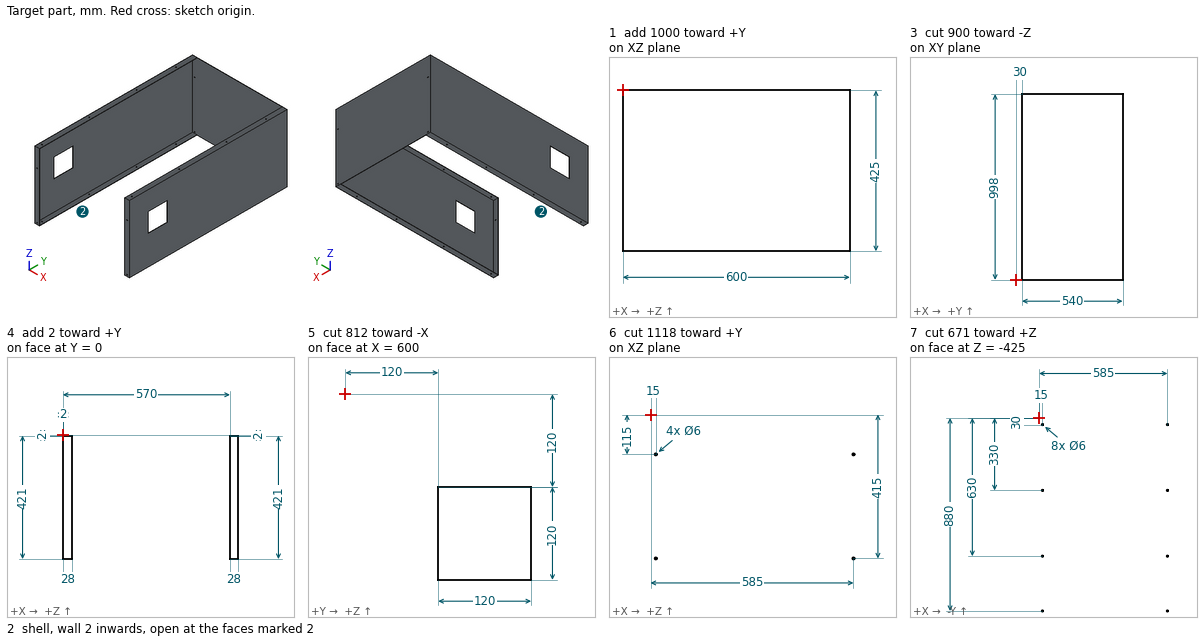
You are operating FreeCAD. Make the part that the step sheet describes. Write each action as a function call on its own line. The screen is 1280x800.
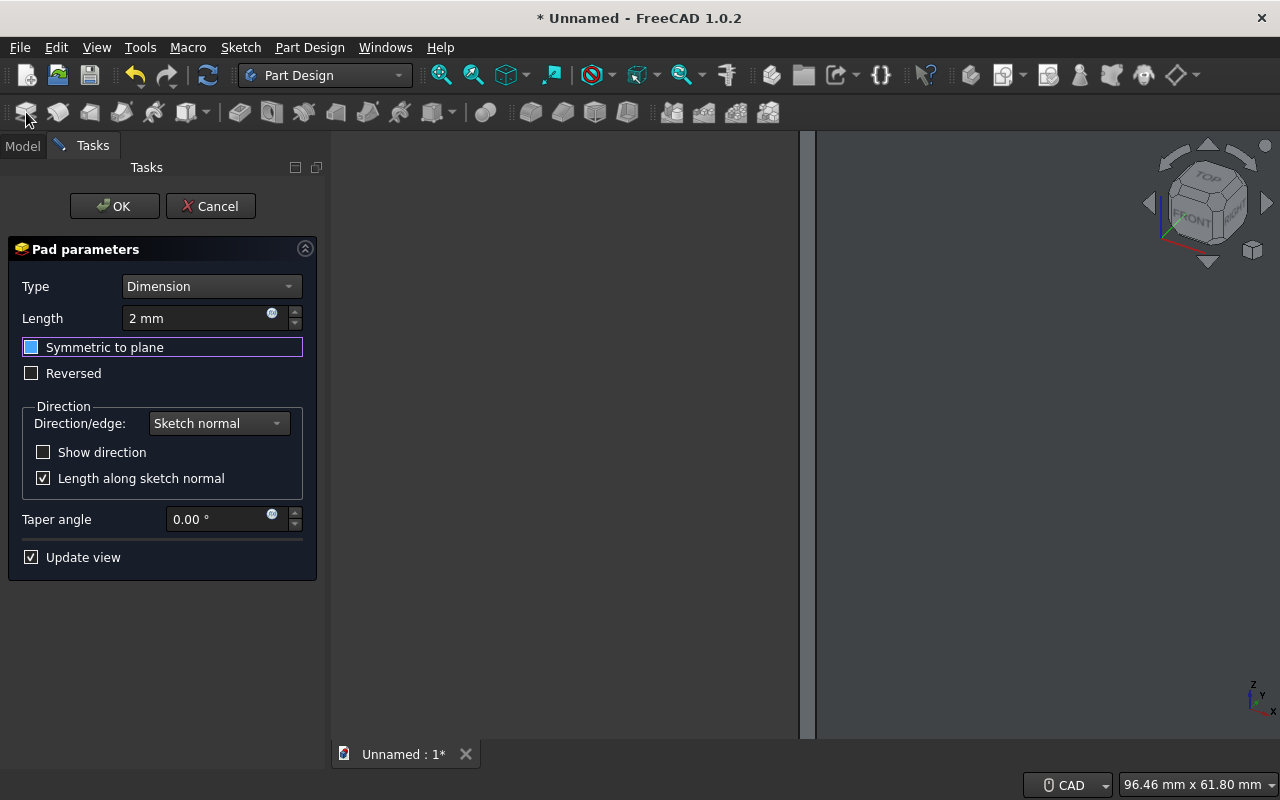
click(30, 373)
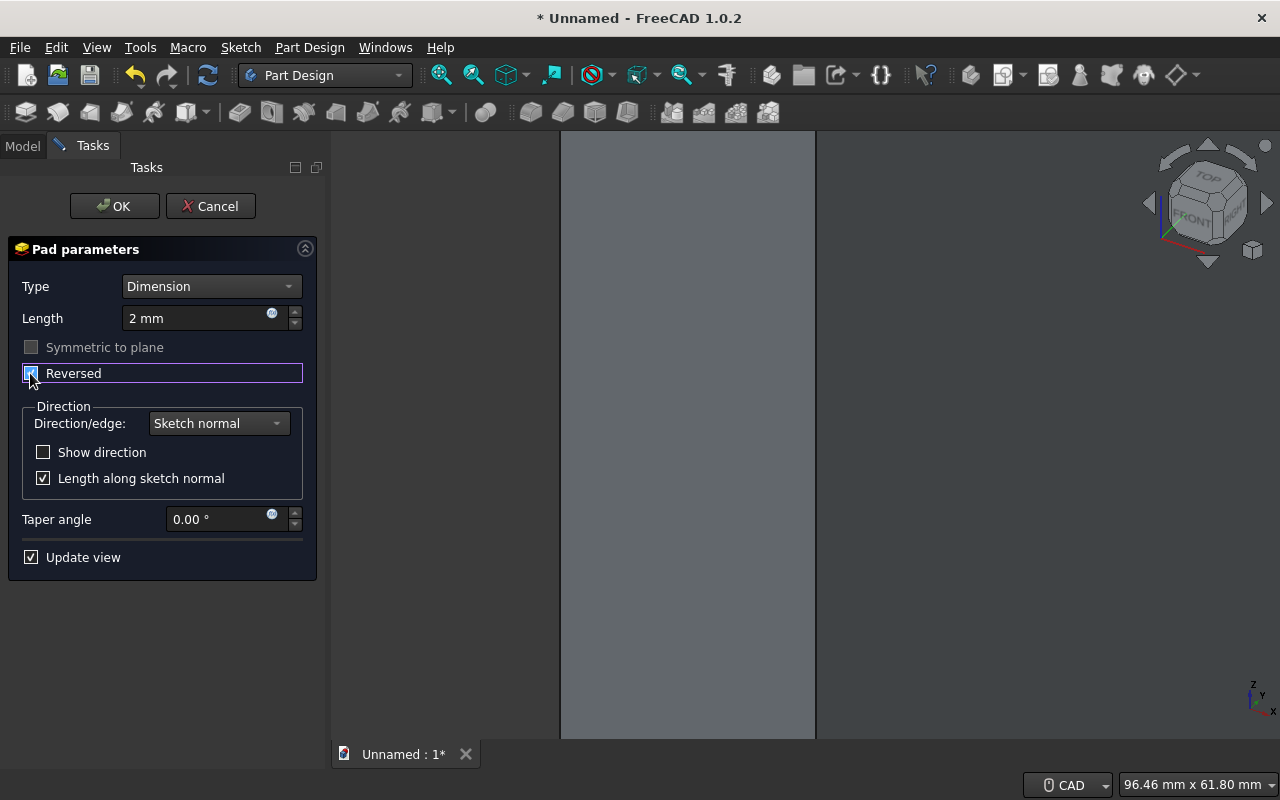
click(115, 206)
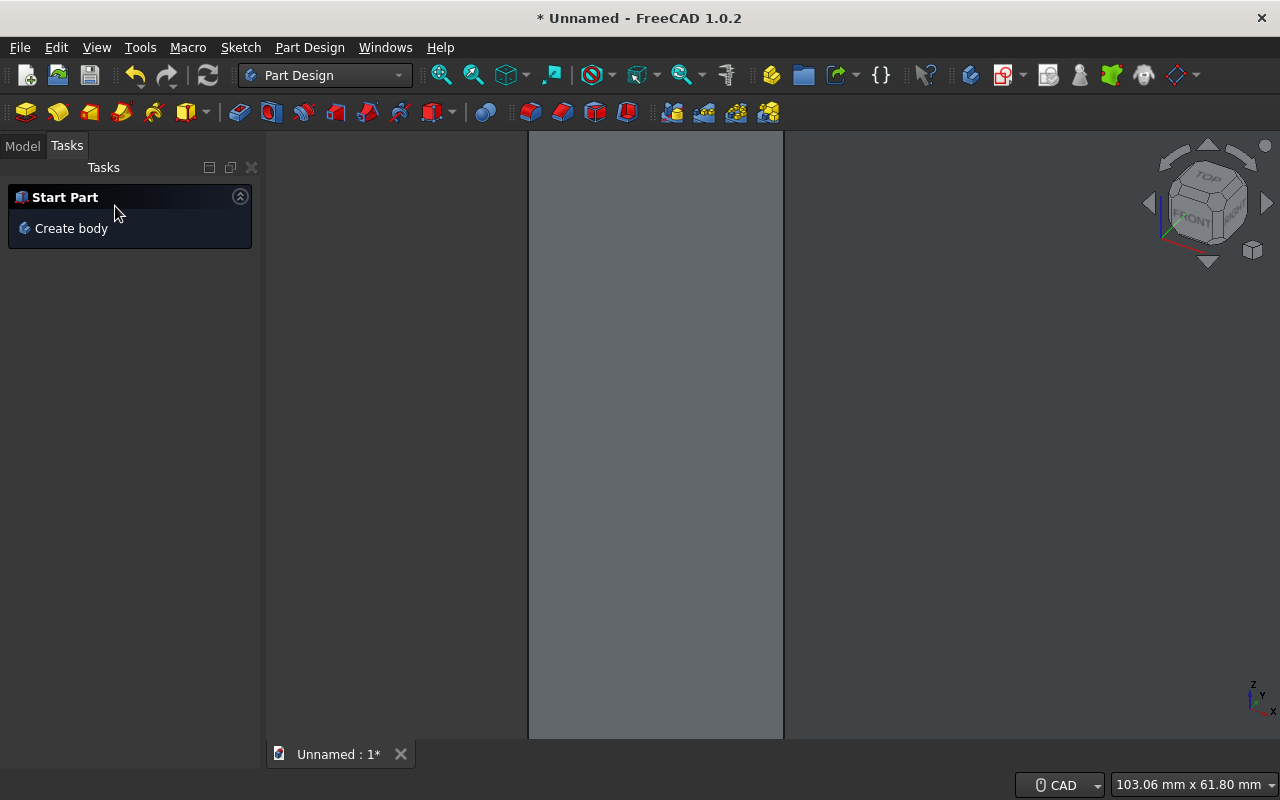
click(442, 76)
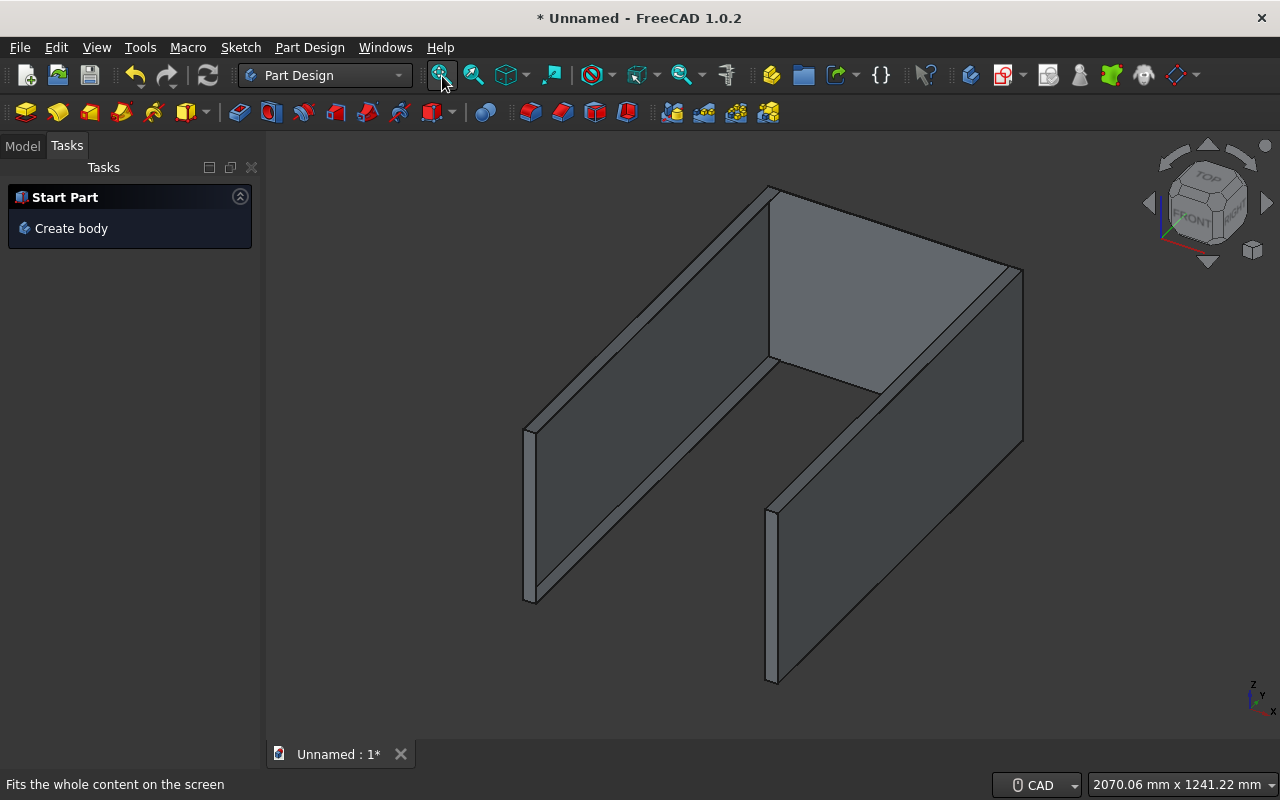
click(970, 407)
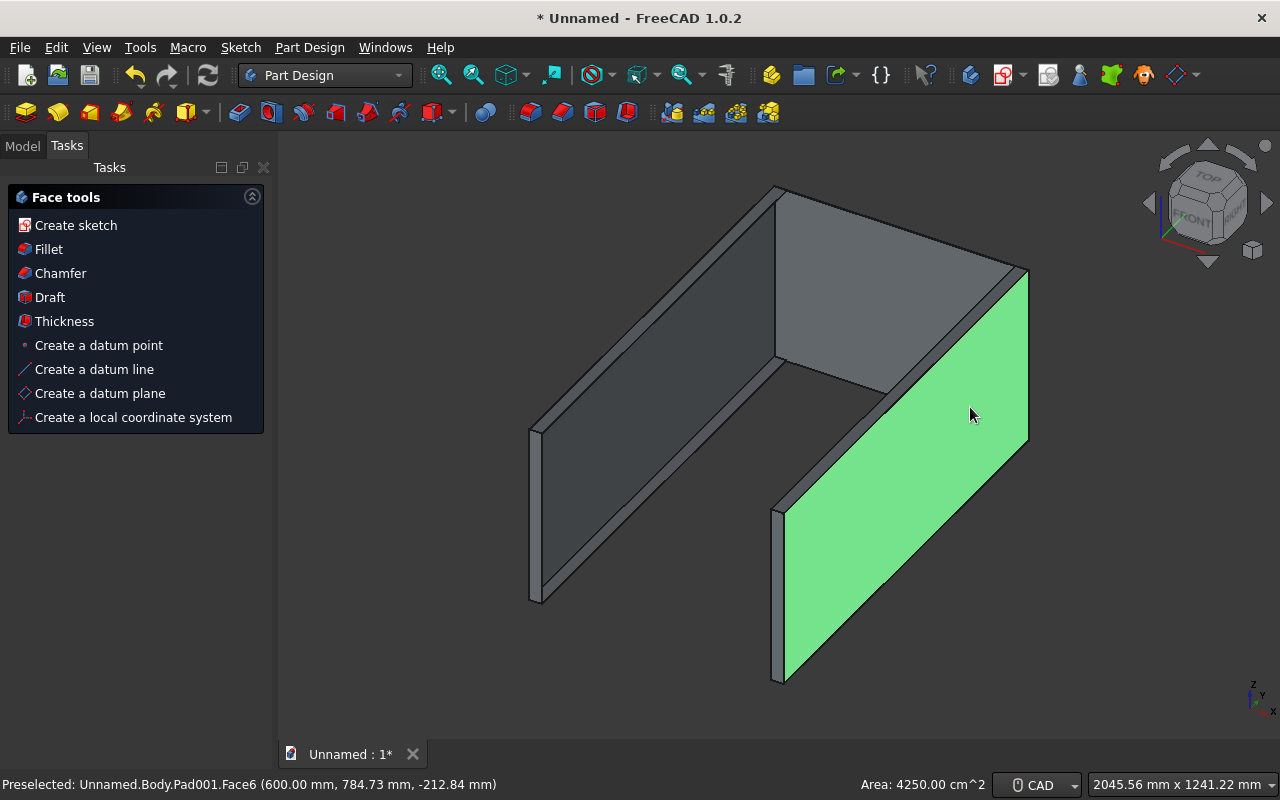
click(1004, 76)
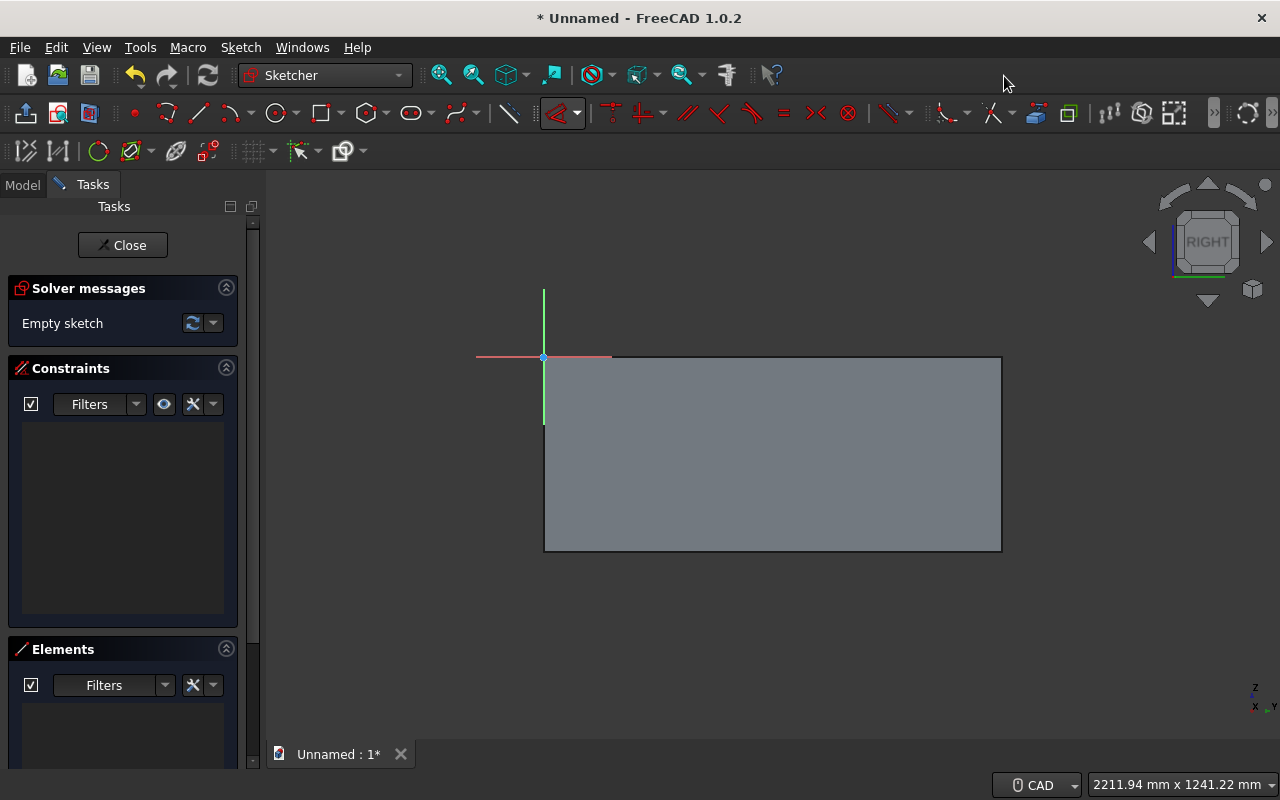
scroll(553, 394, up, 6)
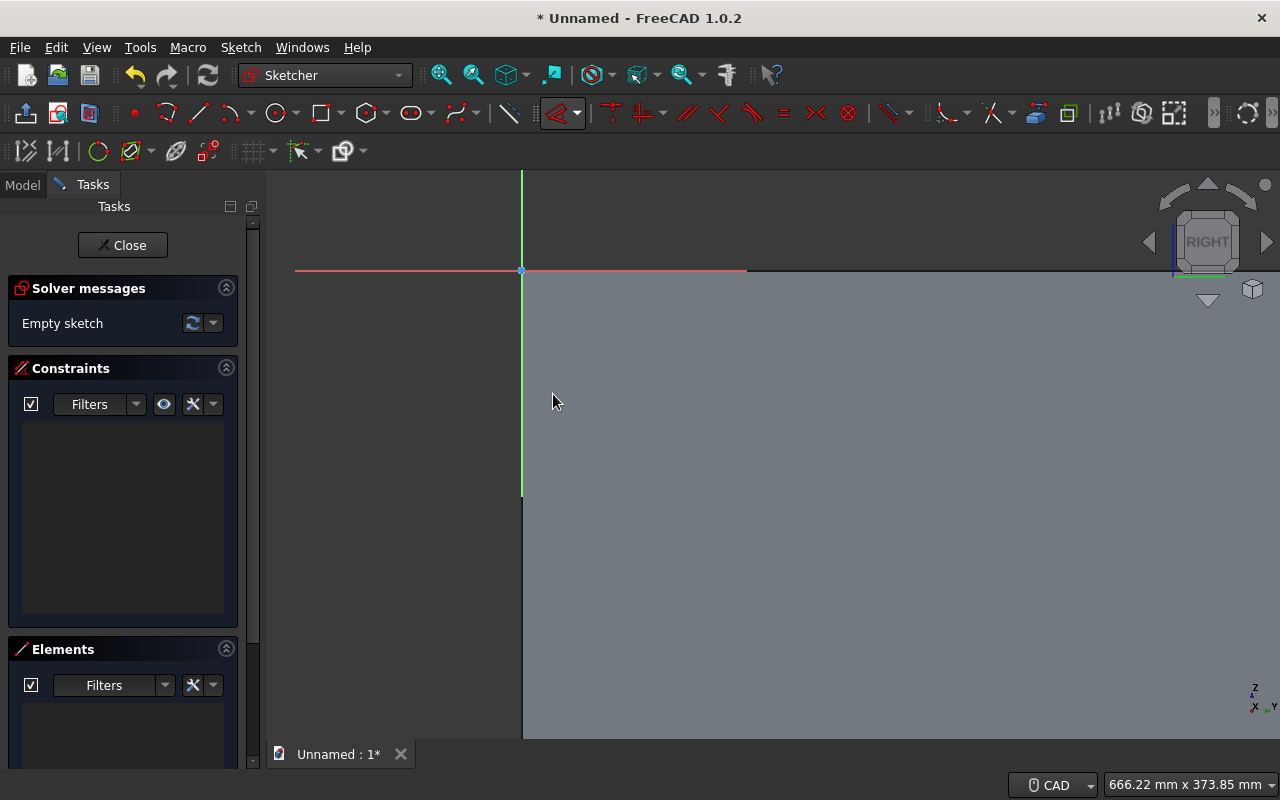
click(322, 114)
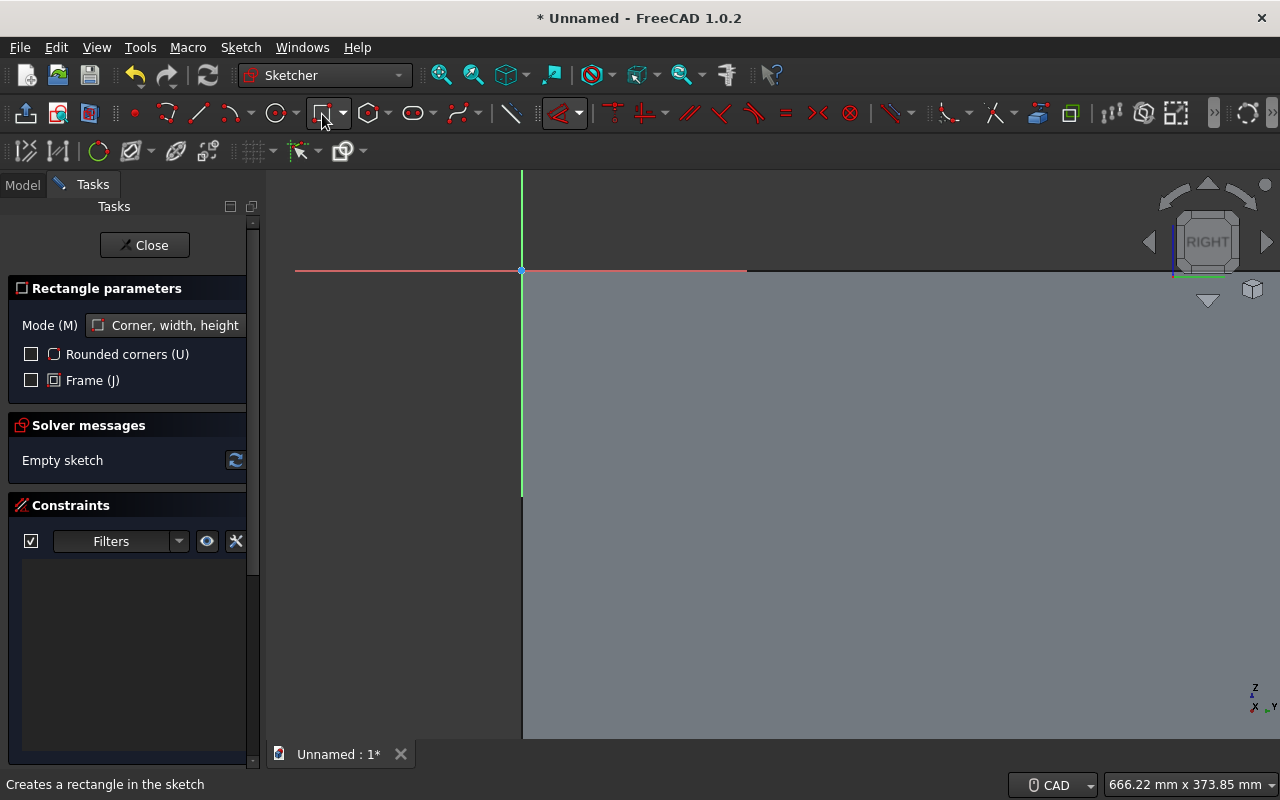
click(704, 453)
move(887, 636)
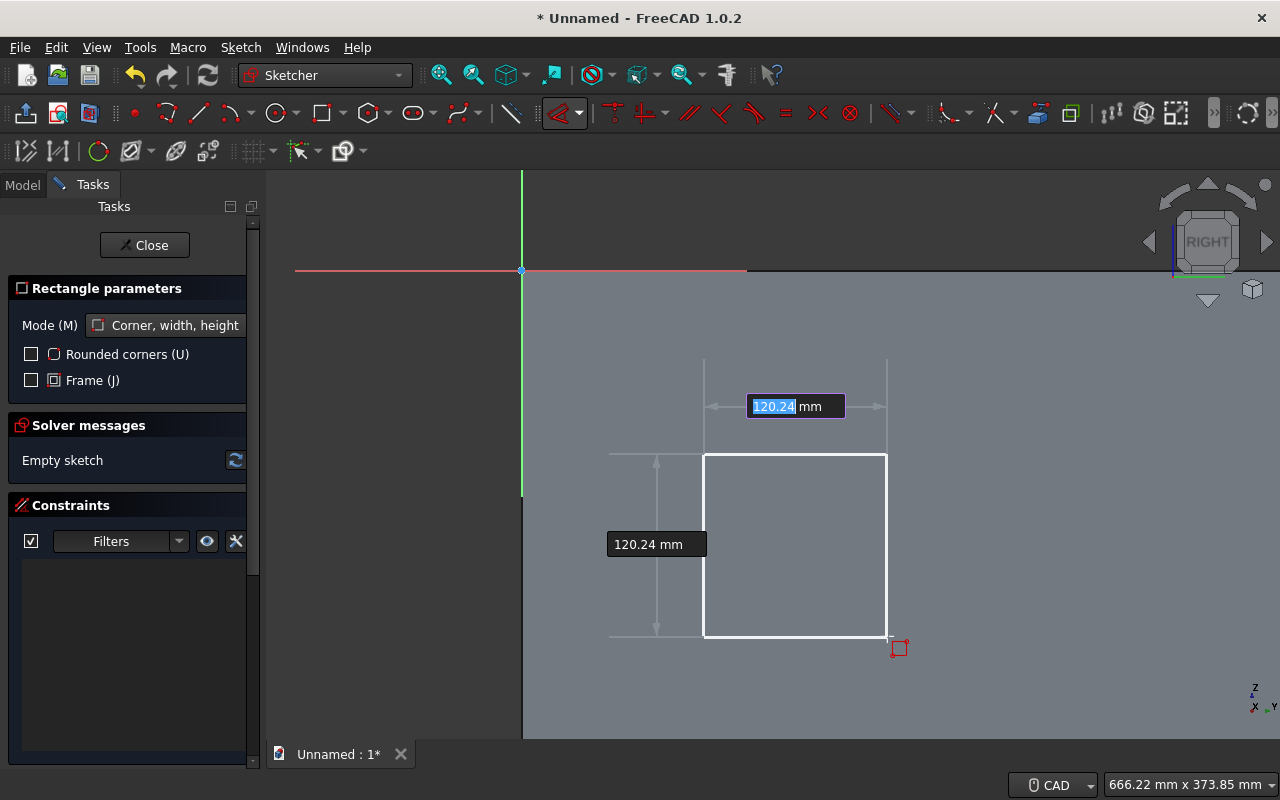
text(120)
key(Tab)
text(120)
key(Return)
key(Escape)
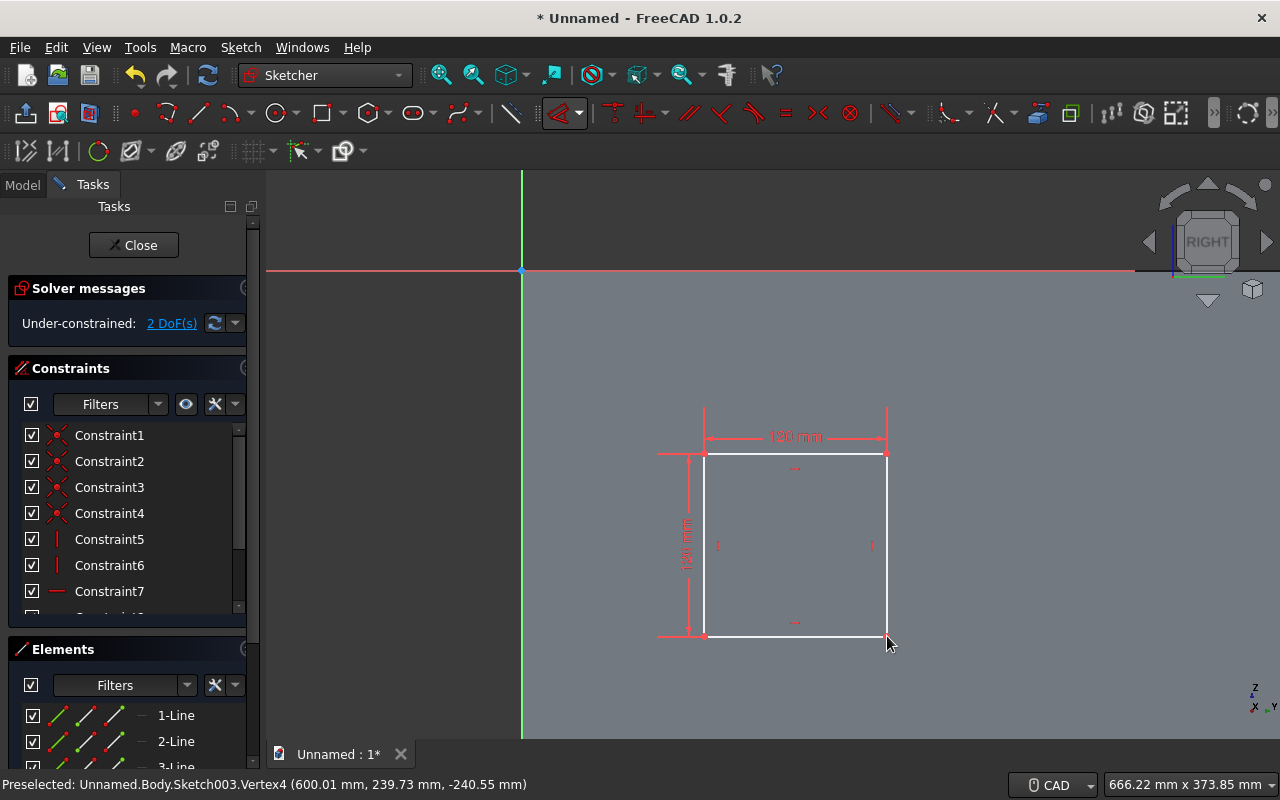
click(704, 454)